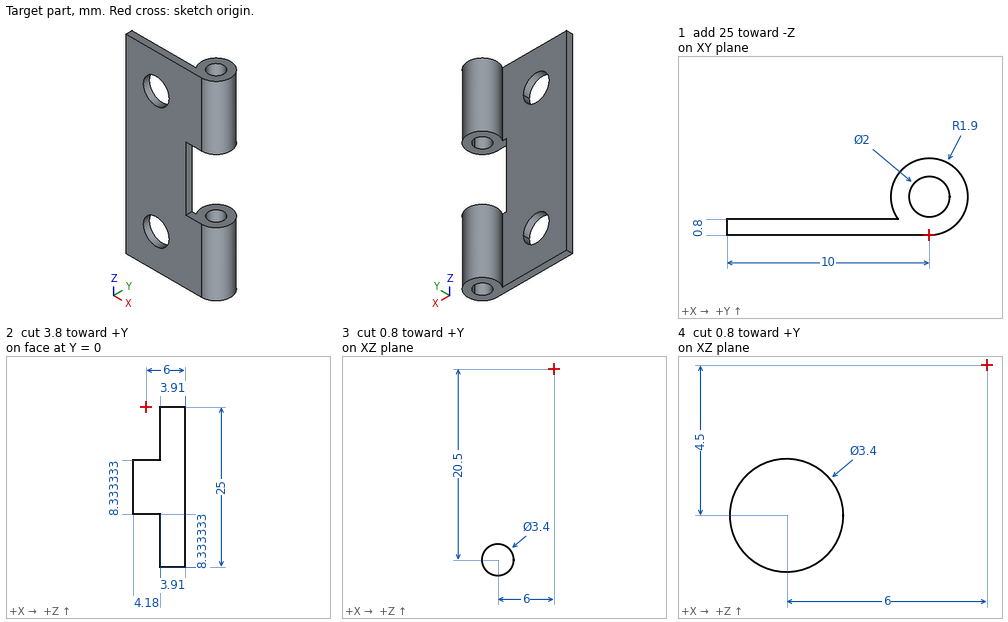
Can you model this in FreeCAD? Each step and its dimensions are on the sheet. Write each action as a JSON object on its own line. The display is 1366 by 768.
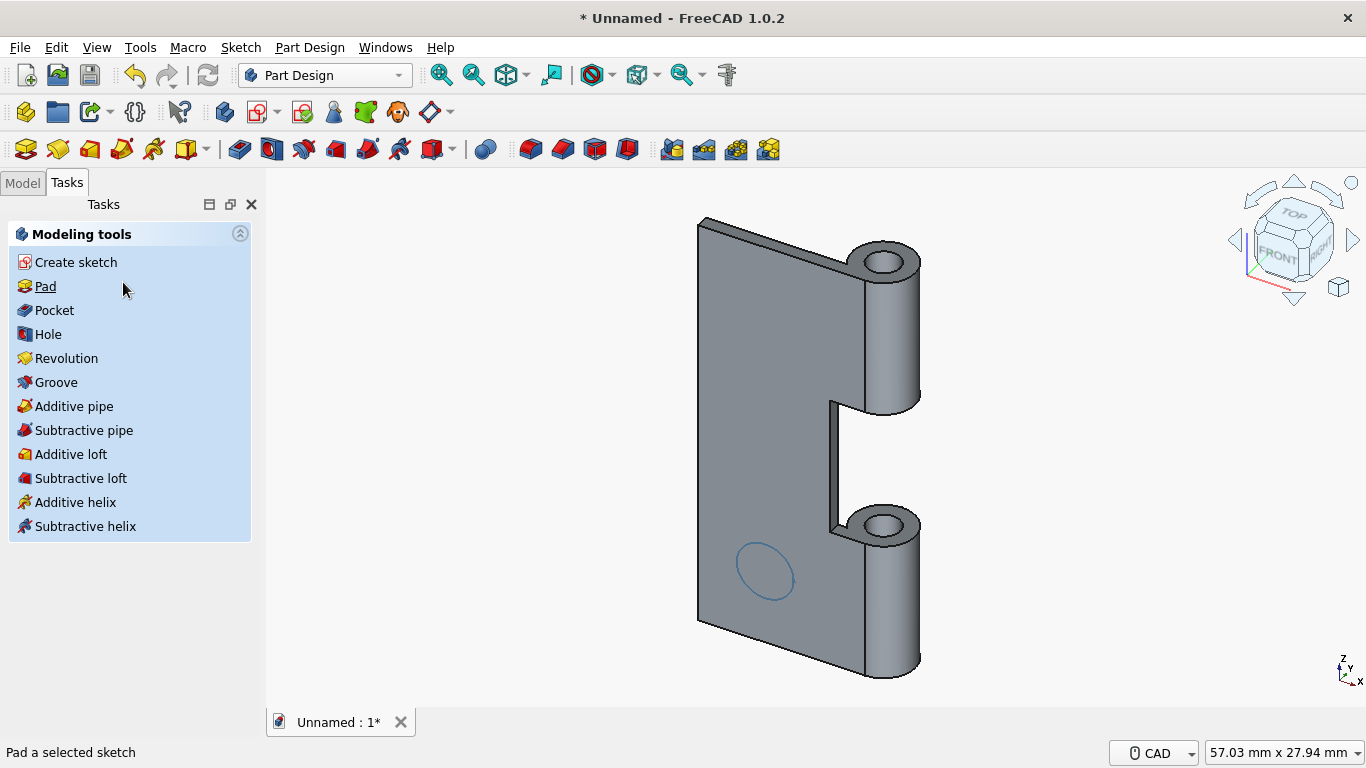
{"action": "left_click", "coordinate": [240, 150]}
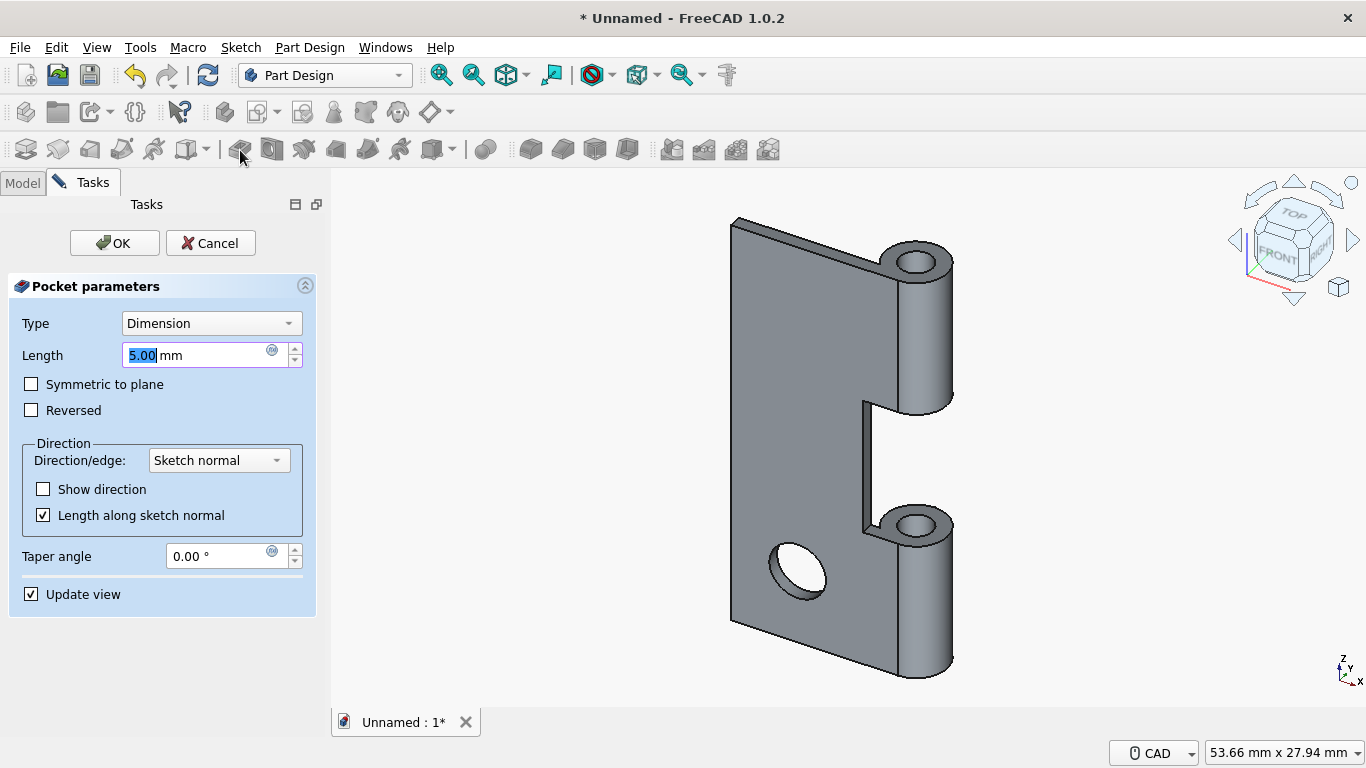
{"action": "type", "text": "0.8"}
{"action": "key", "text": "Tab"}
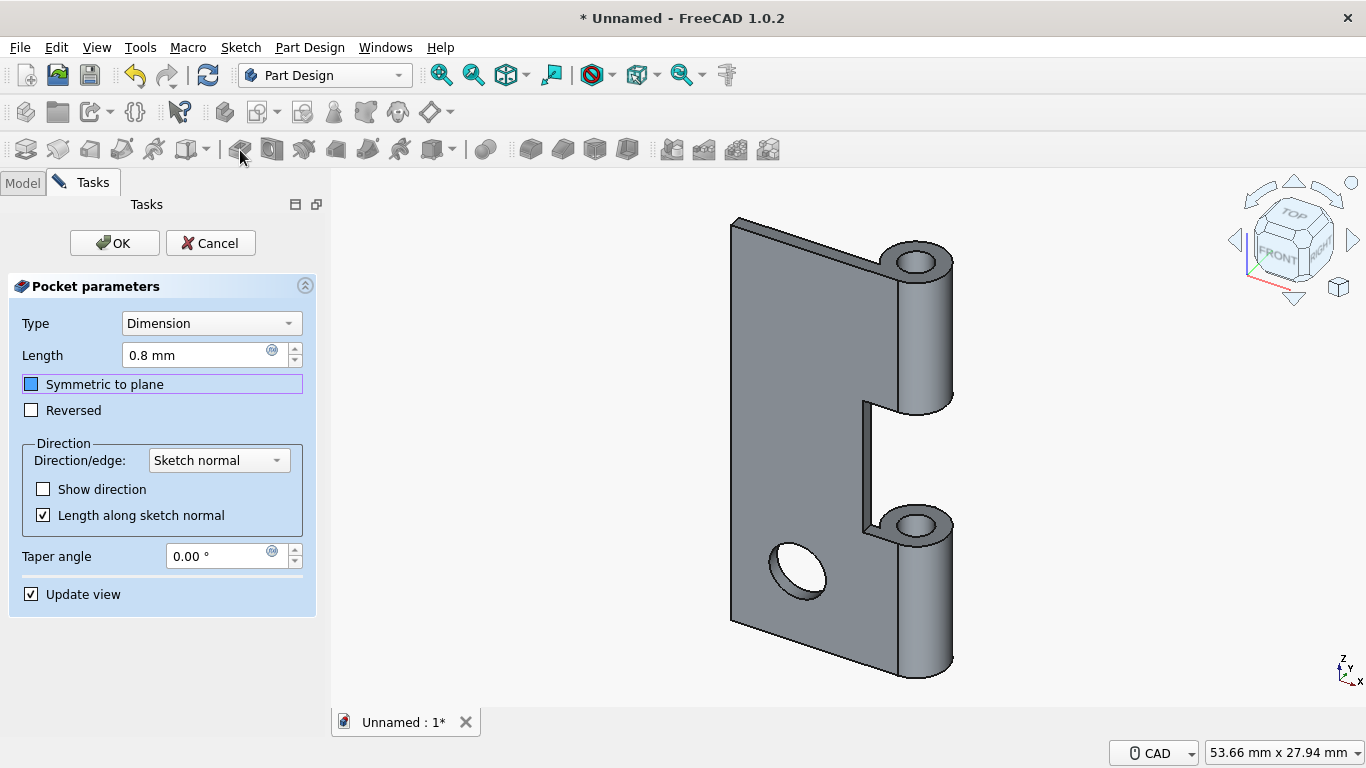
{"action": "left_click", "coordinate": [115, 243]}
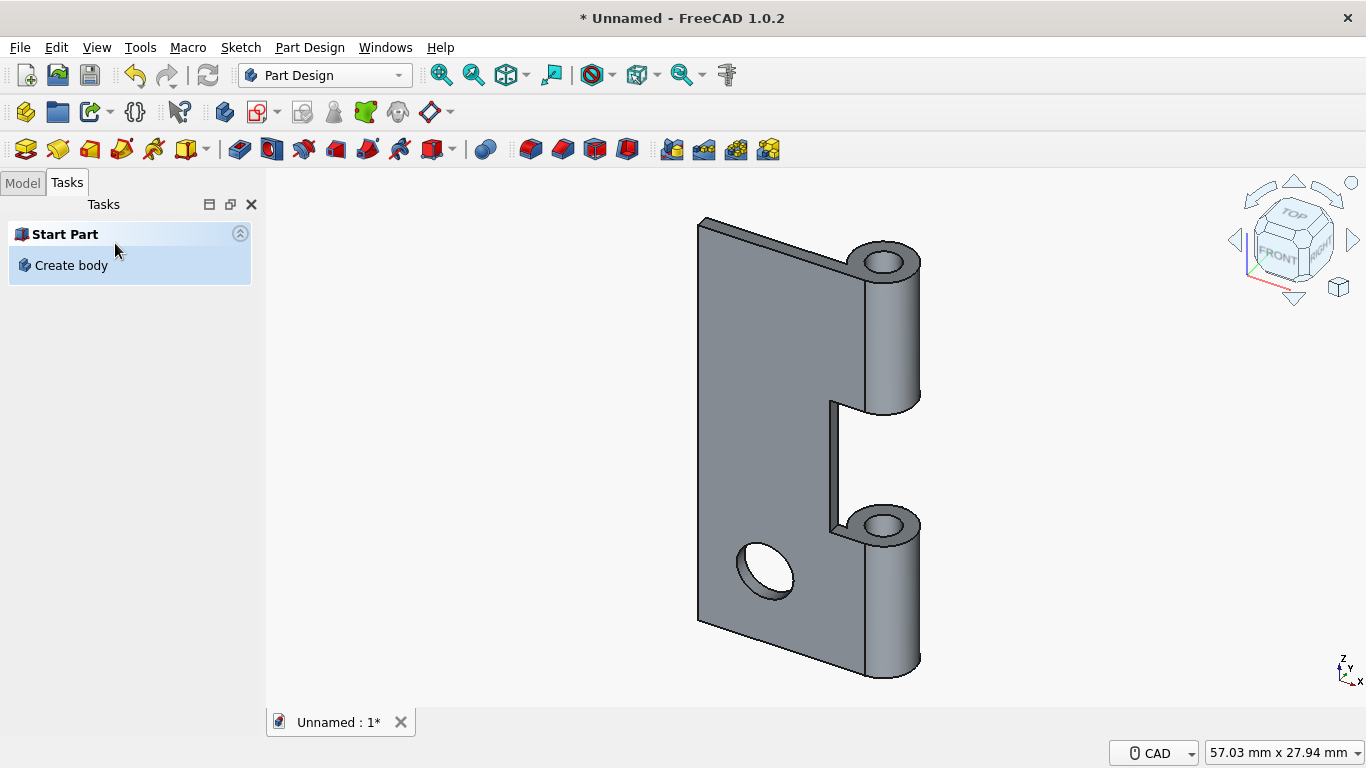
{"action": "left_click", "coordinate": [258, 112]}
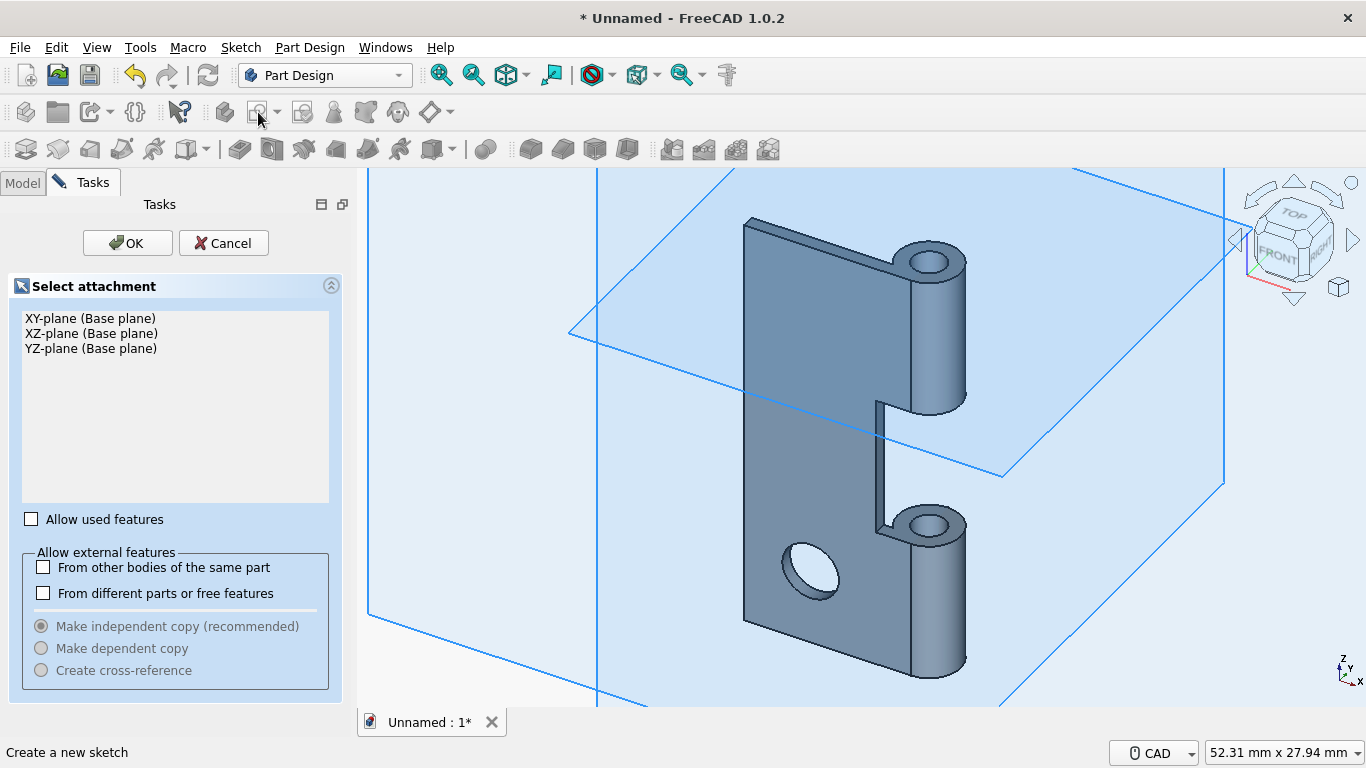
{"action": "left_click", "coordinate": [82, 334]}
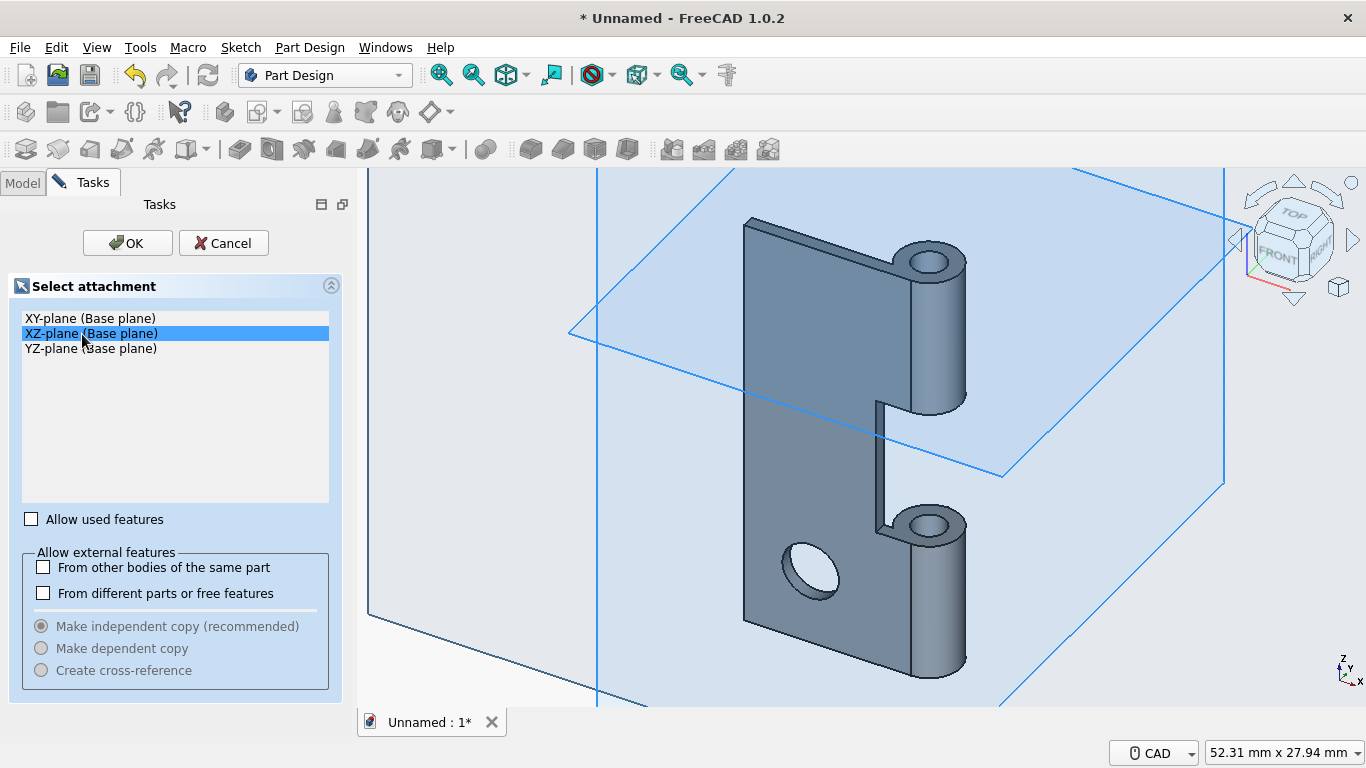
{"action": "left_click", "coordinate": [128, 243]}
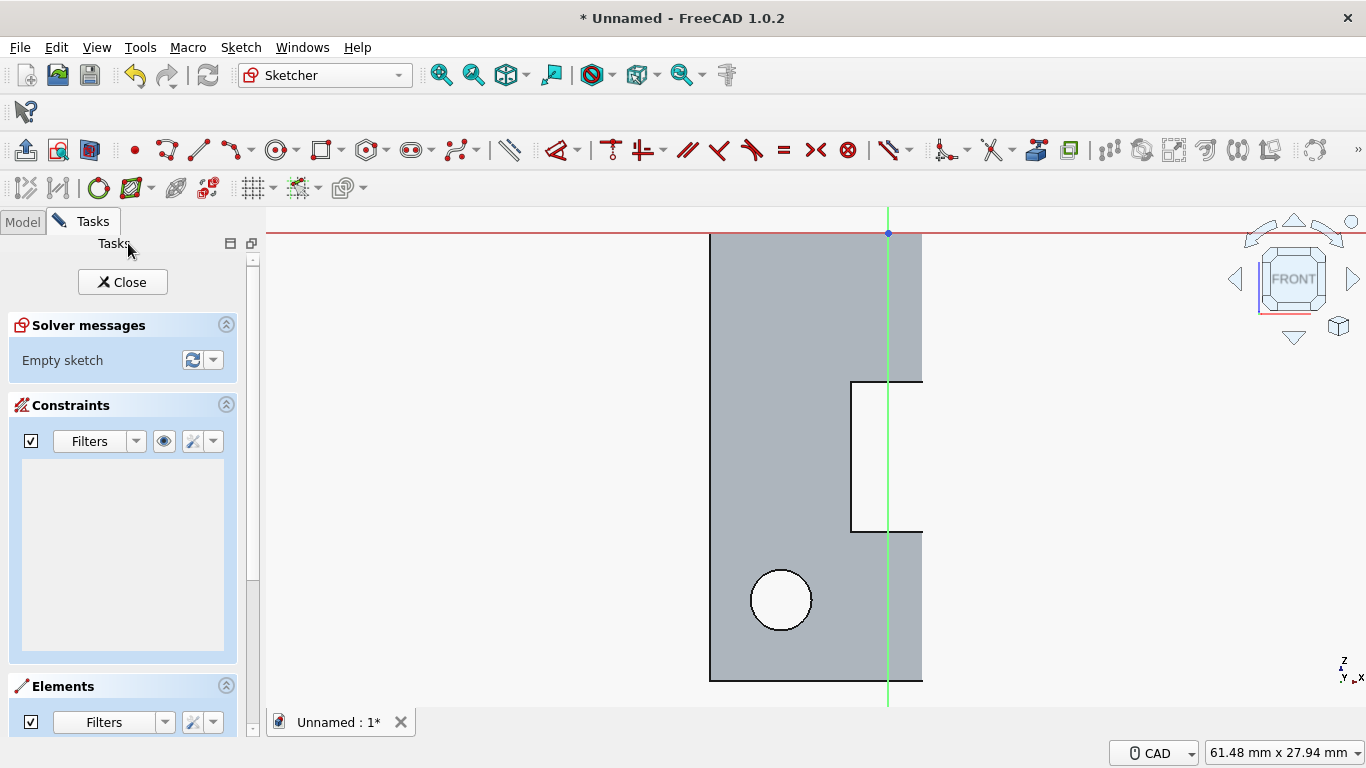
{"action": "scroll", "coordinate": [748, 457], "scroll_direction": "down", "scroll_amount": 5}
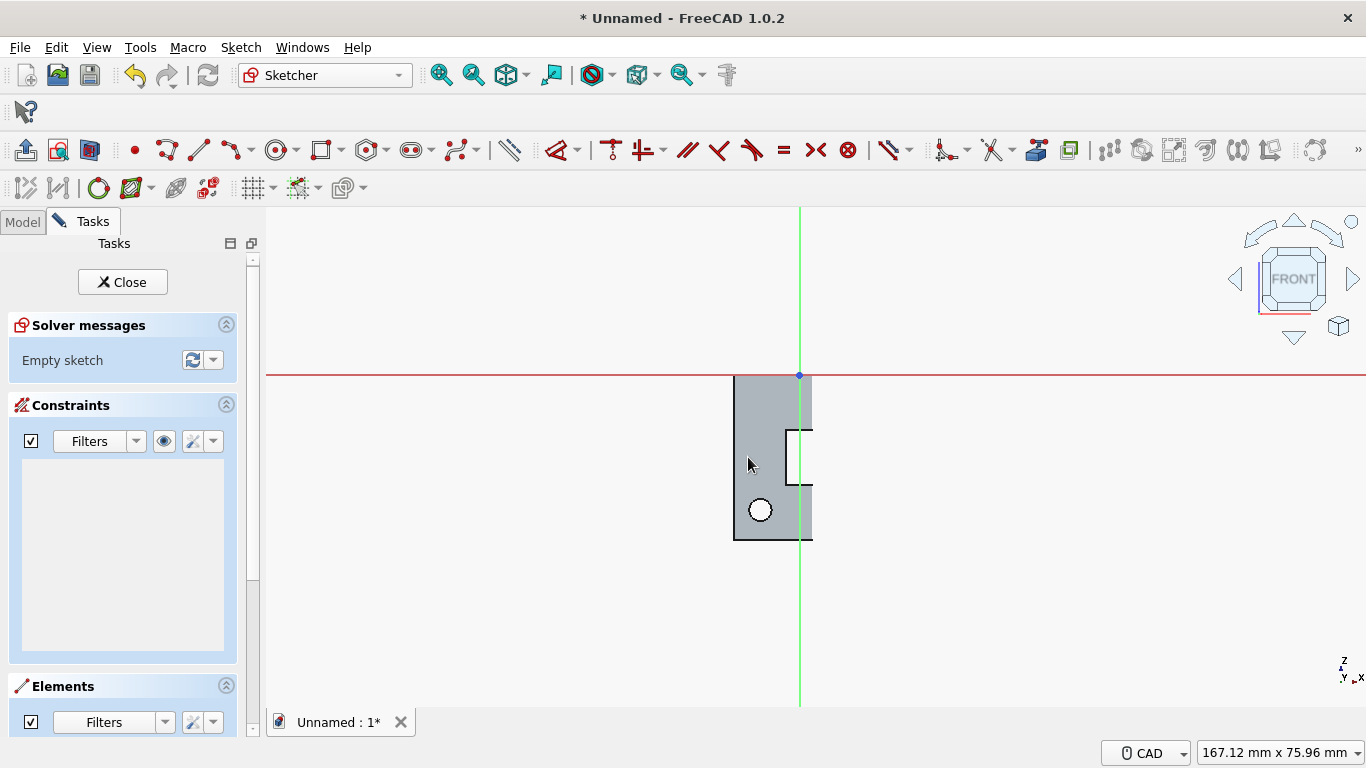
{"action": "scroll", "coordinate": [779, 386], "scroll_direction": "up", "scroll_amount": 10}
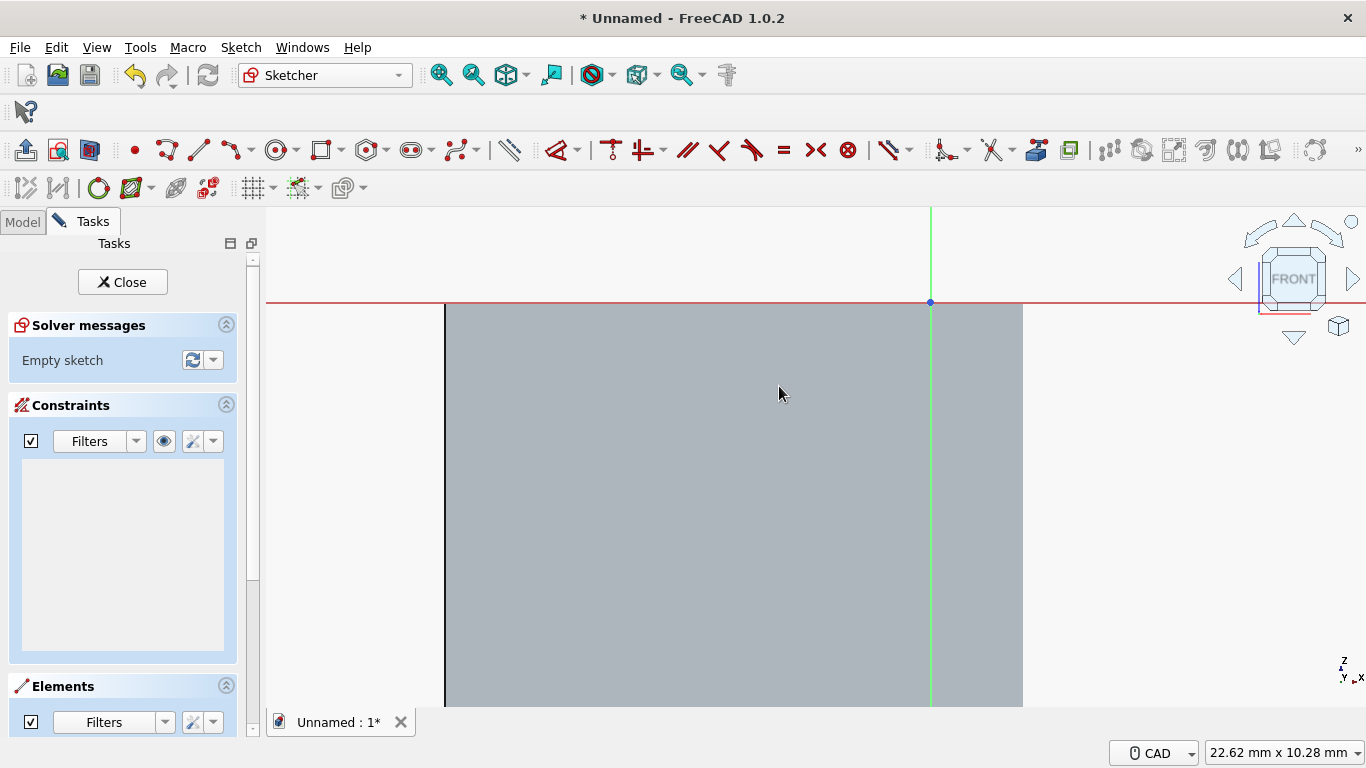
{"action": "left_click", "coordinate": [276, 150]}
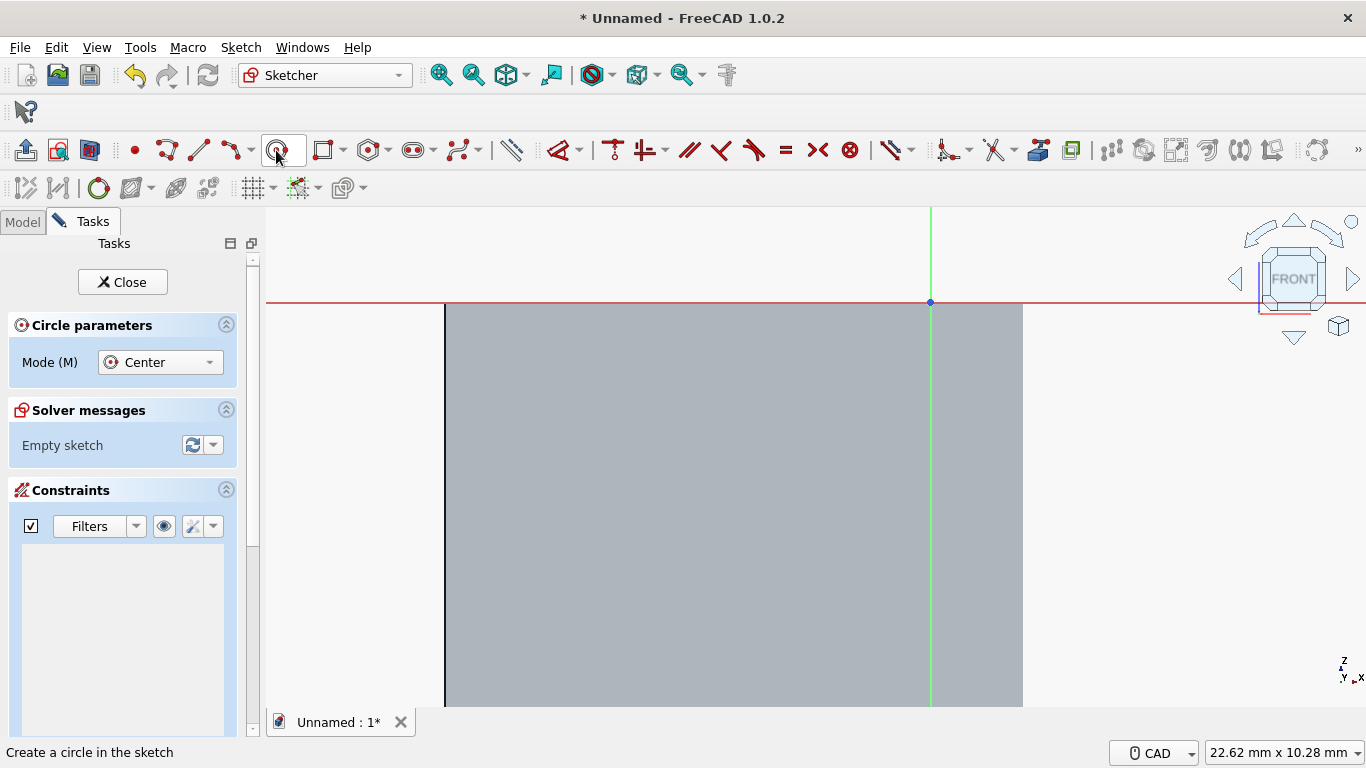
{"action": "left_click", "coordinate": [639, 522]}
{"action": "left_click", "coordinate": [698, 463]}
{"action": "key", "text": "Escape"}